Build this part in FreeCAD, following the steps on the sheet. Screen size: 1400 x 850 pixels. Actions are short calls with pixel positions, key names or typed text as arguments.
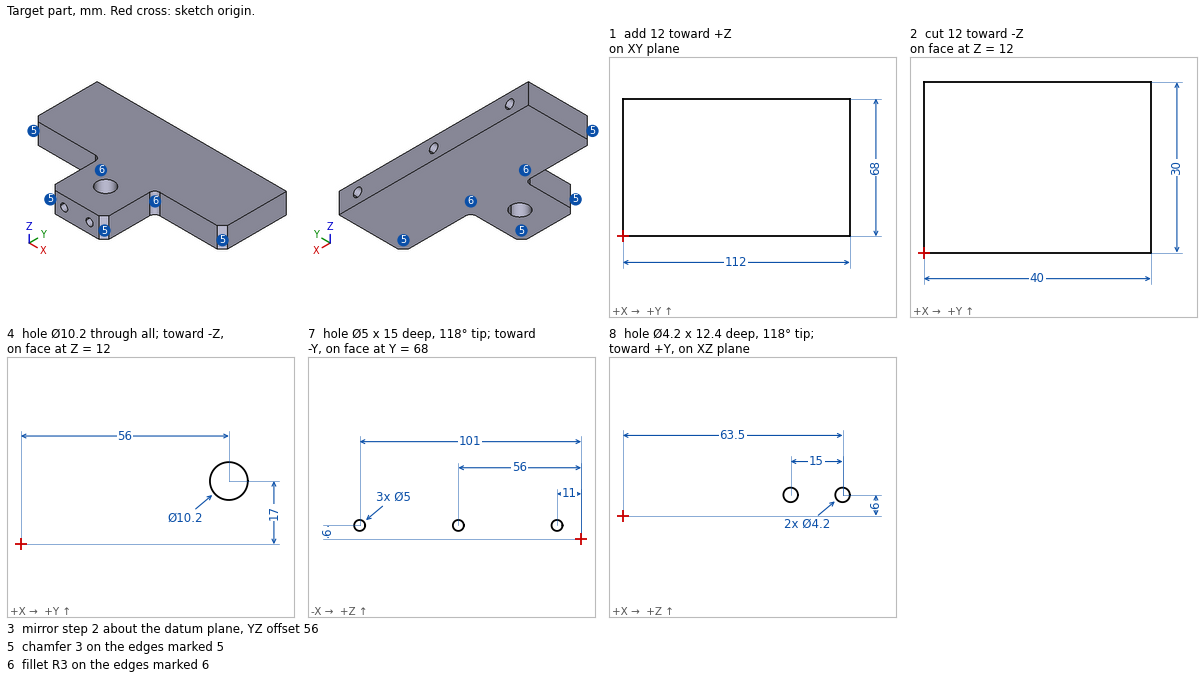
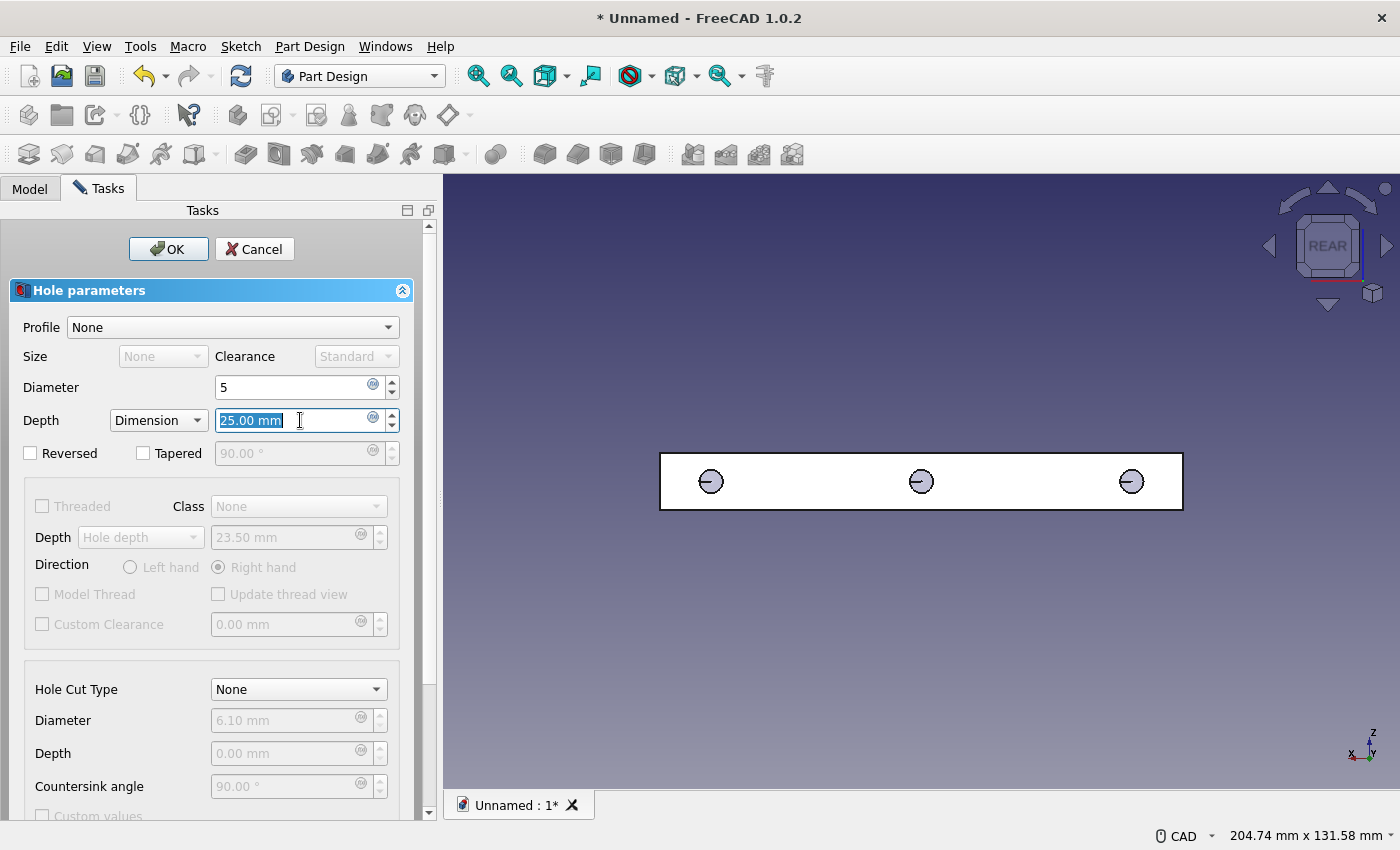
text(15)
key(Tab)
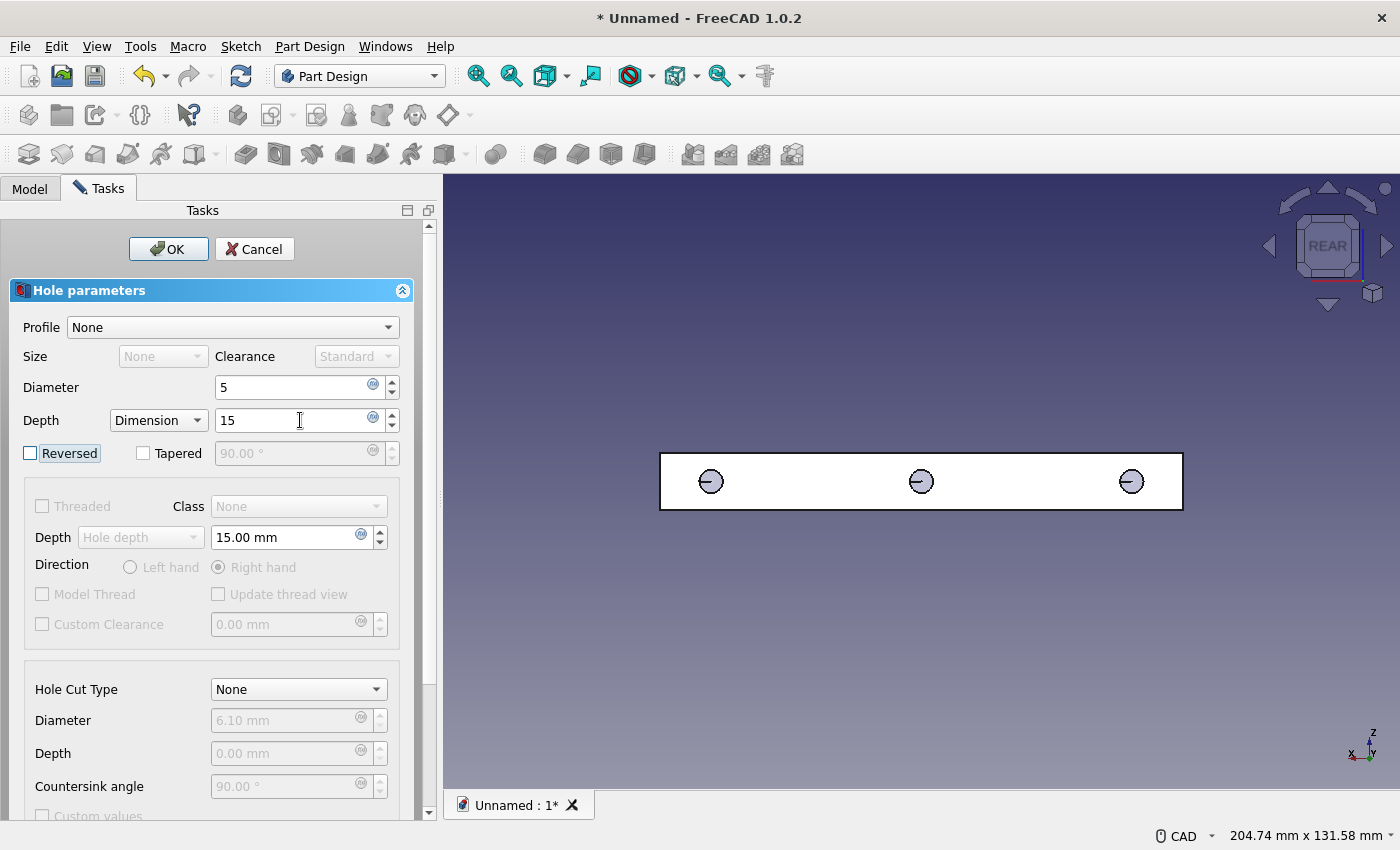
click(169, 249)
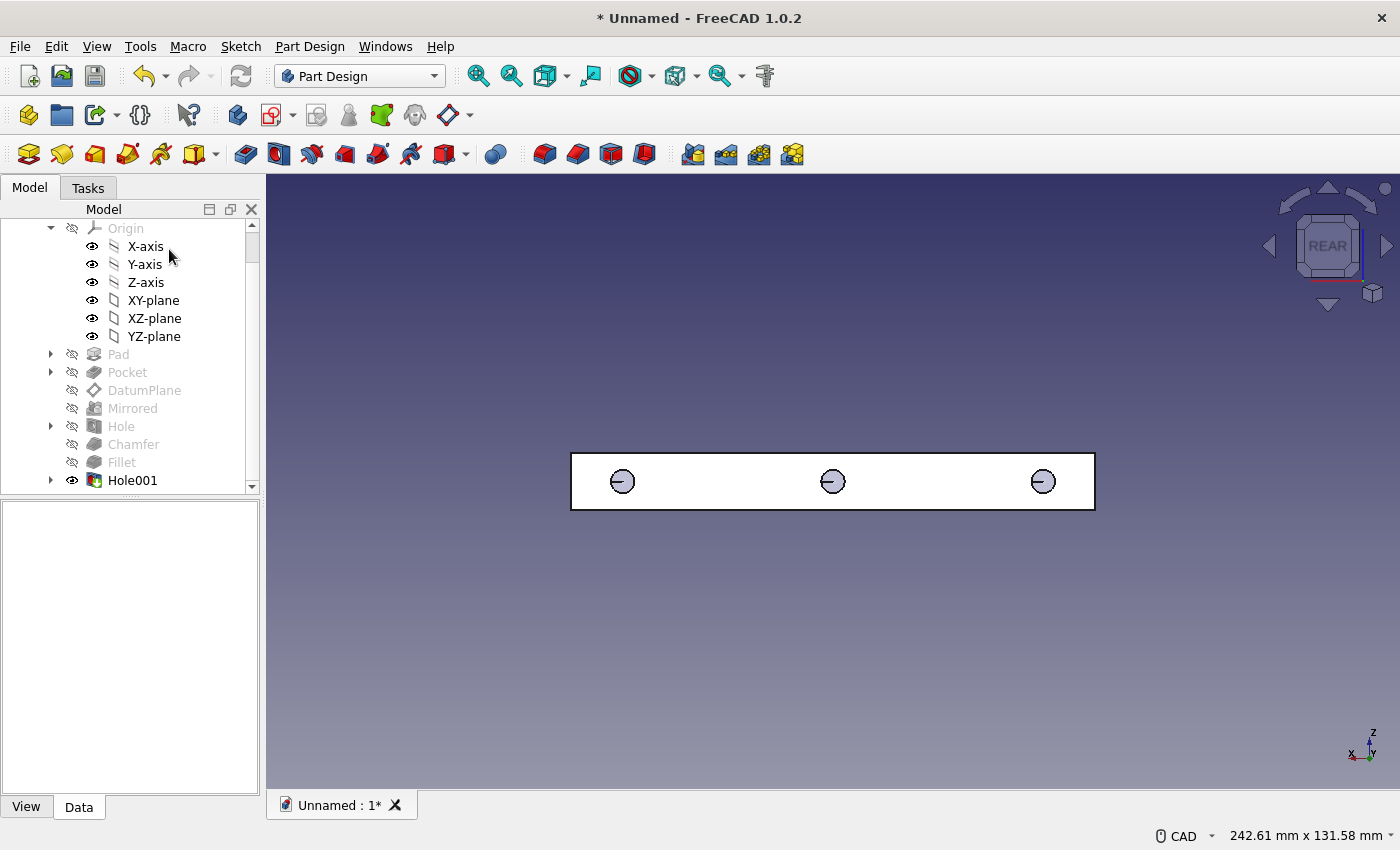
click(270, 116)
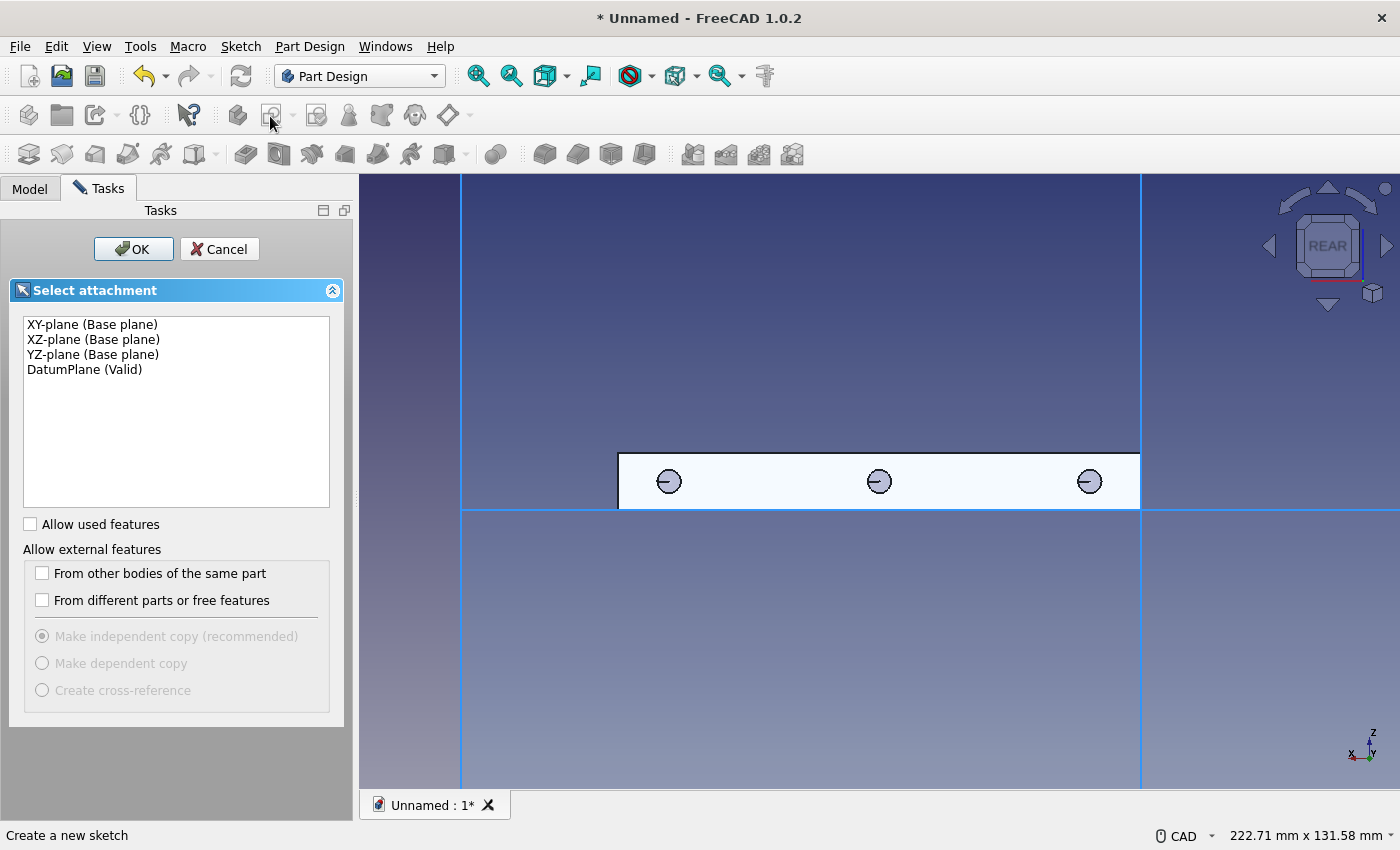
click(84, 340)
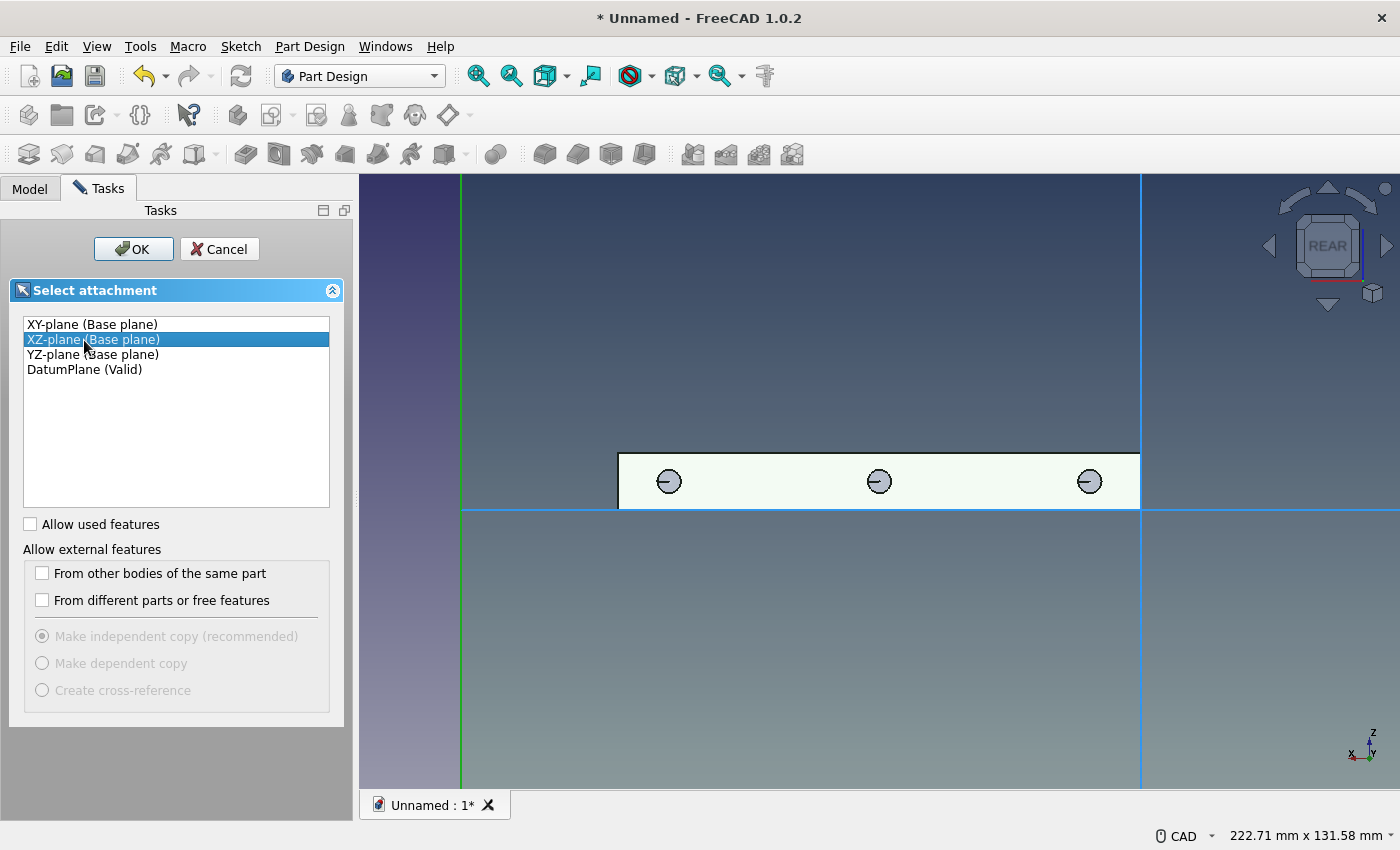
click(134, 249)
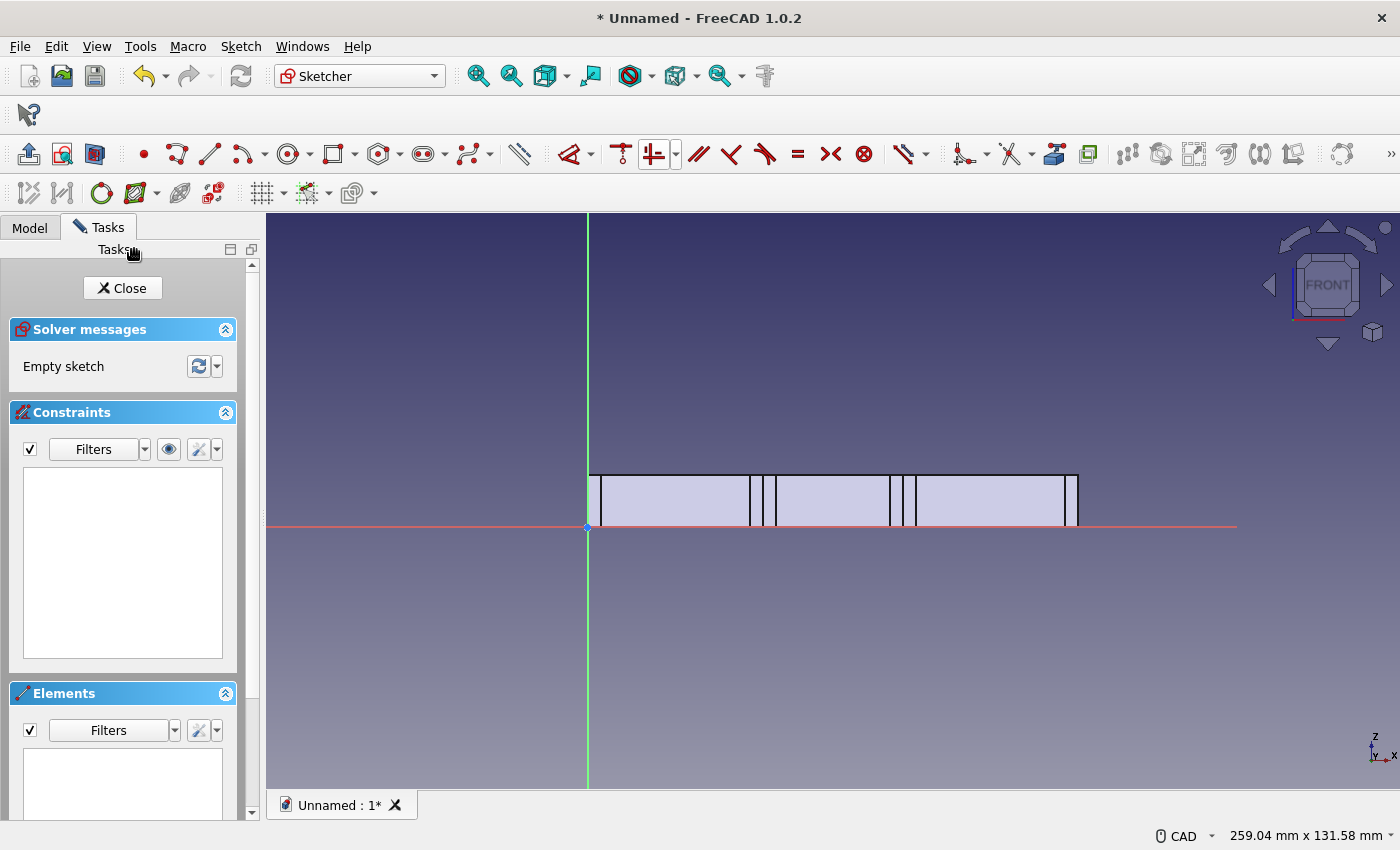
scroll(844, 501, up, 10)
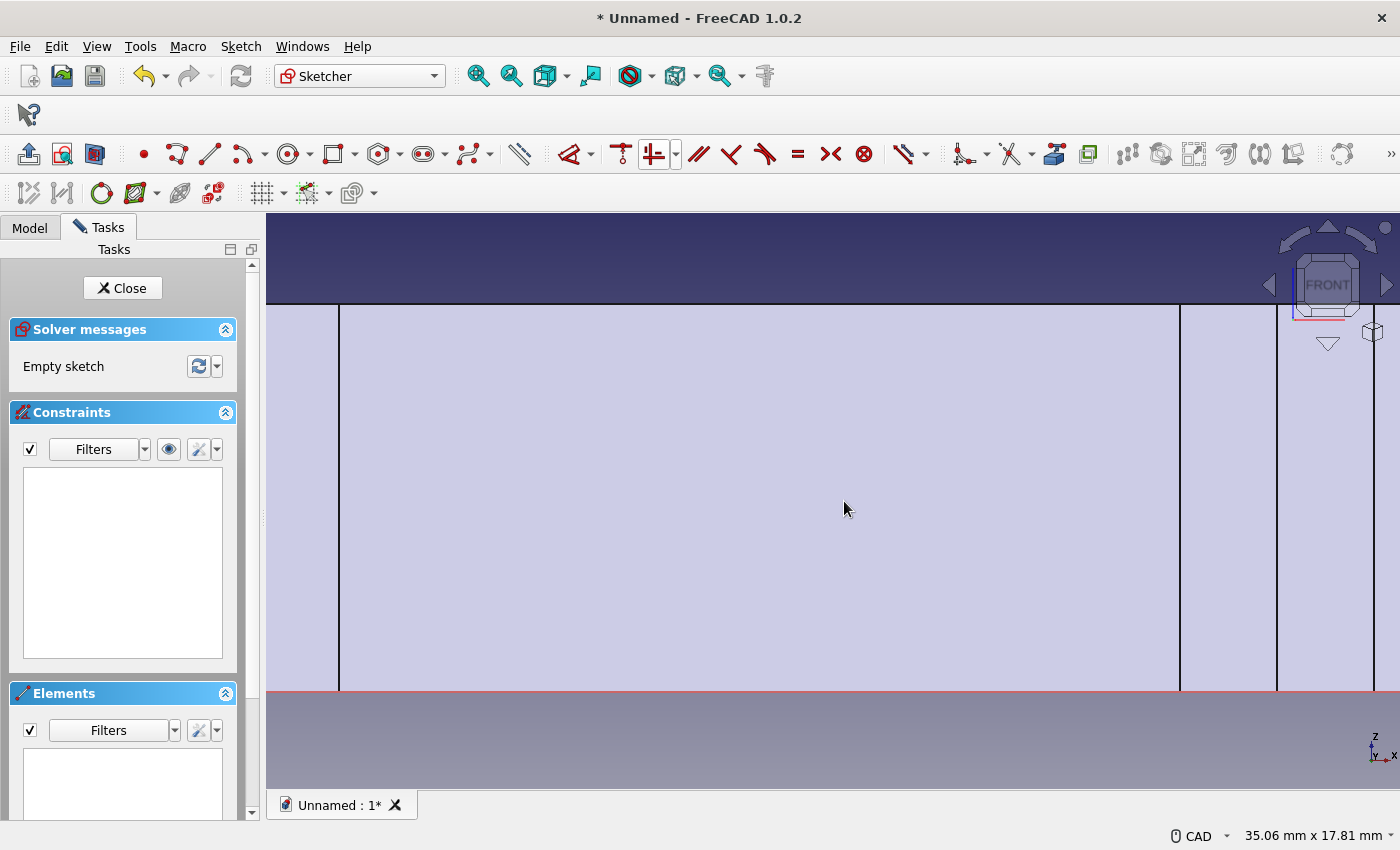
click(288, 154)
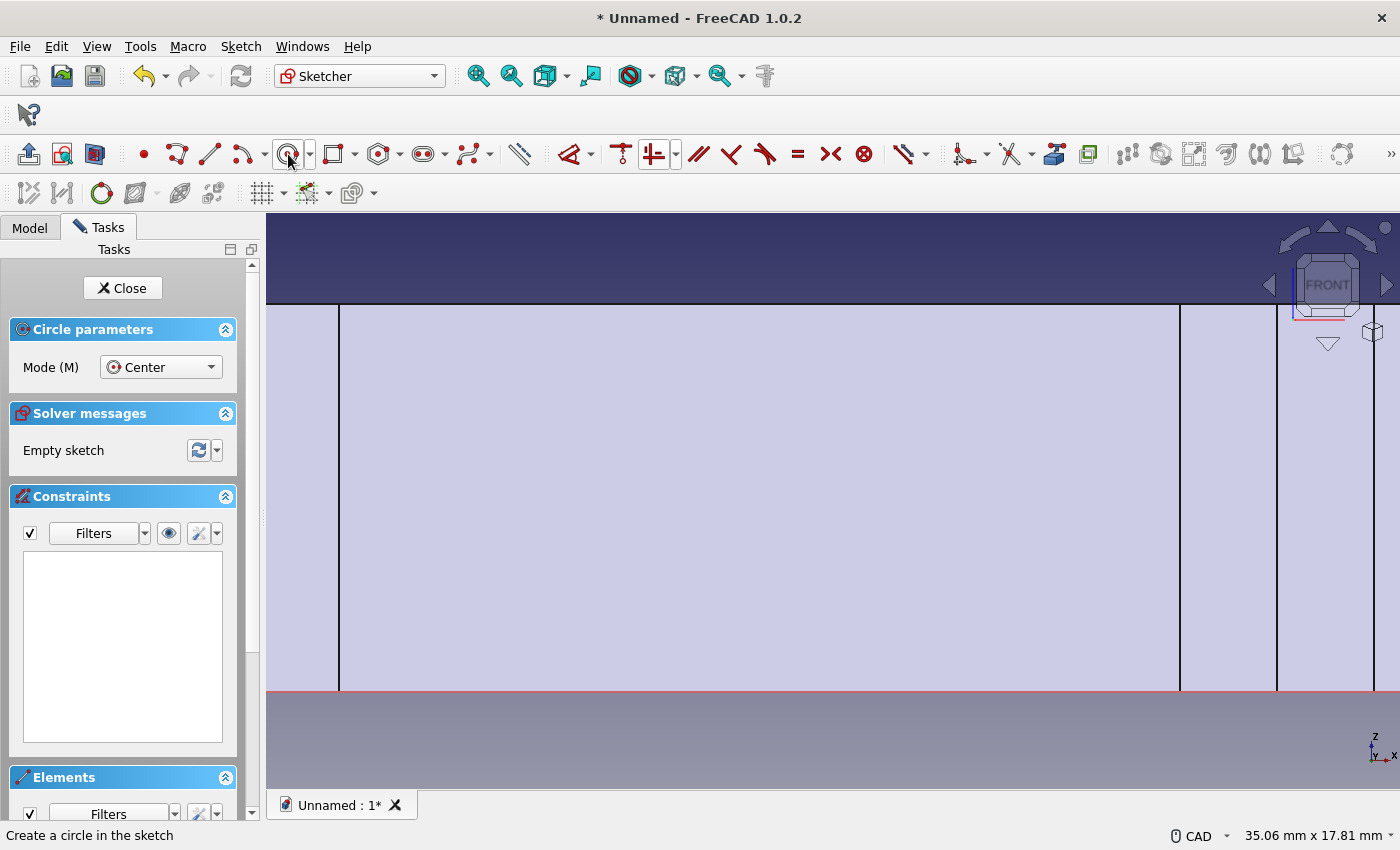
click(1002, 498)
click(1050, 450)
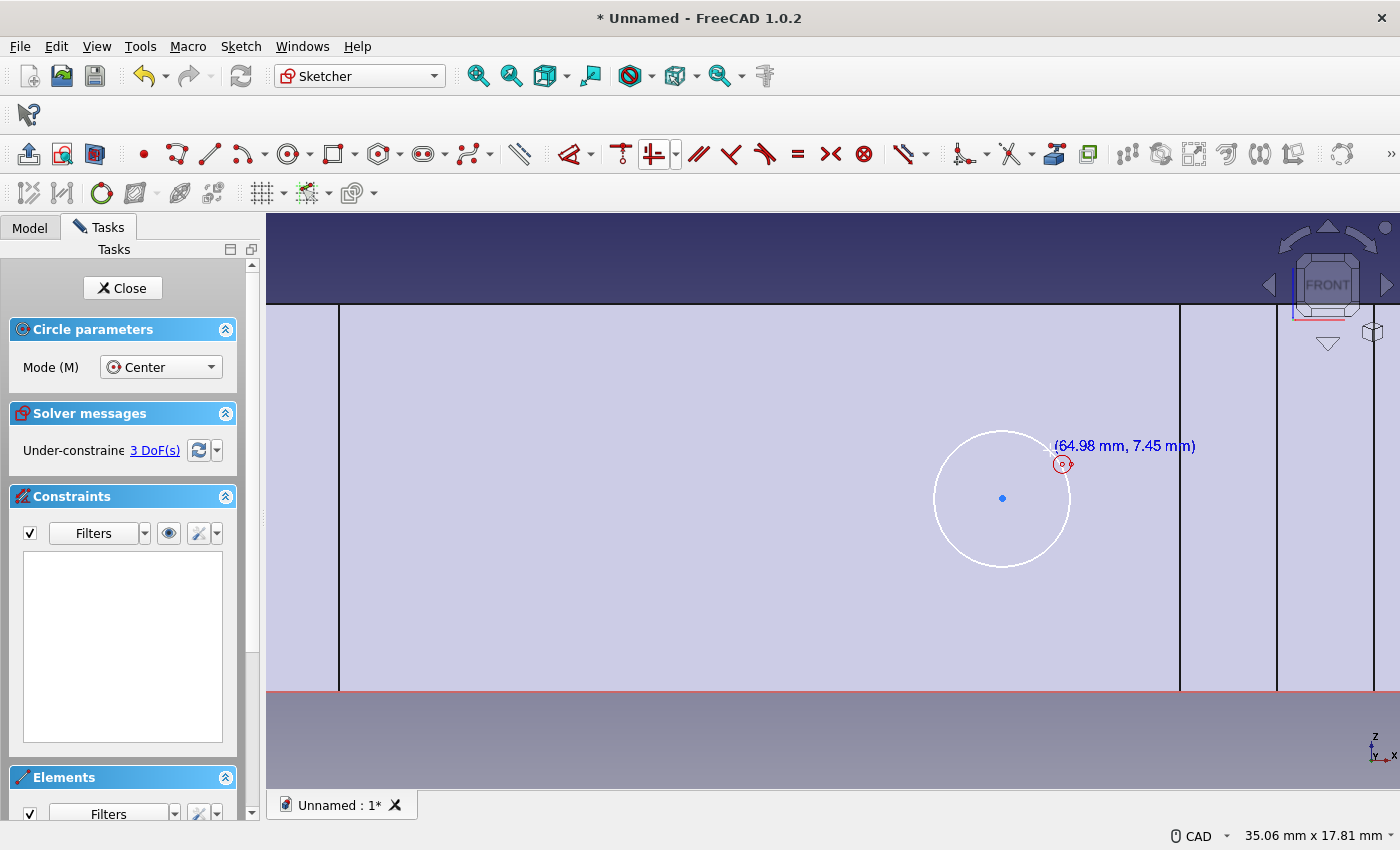
click(517, 498)
click(565, 450)
key(Escape)